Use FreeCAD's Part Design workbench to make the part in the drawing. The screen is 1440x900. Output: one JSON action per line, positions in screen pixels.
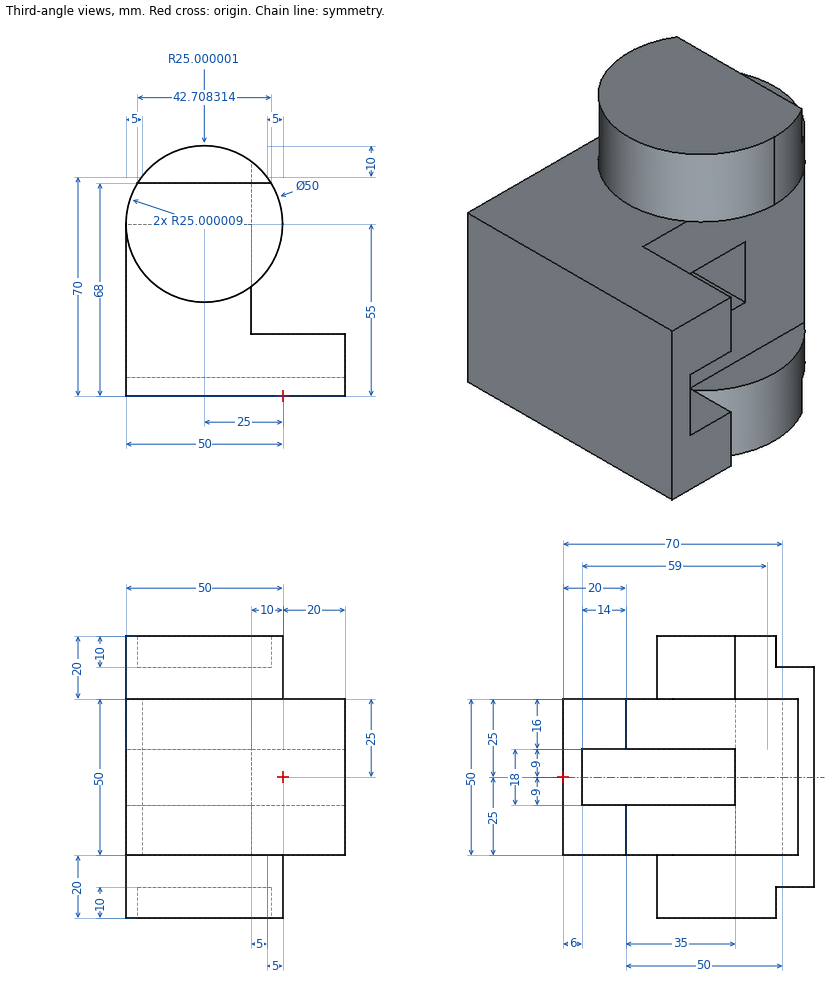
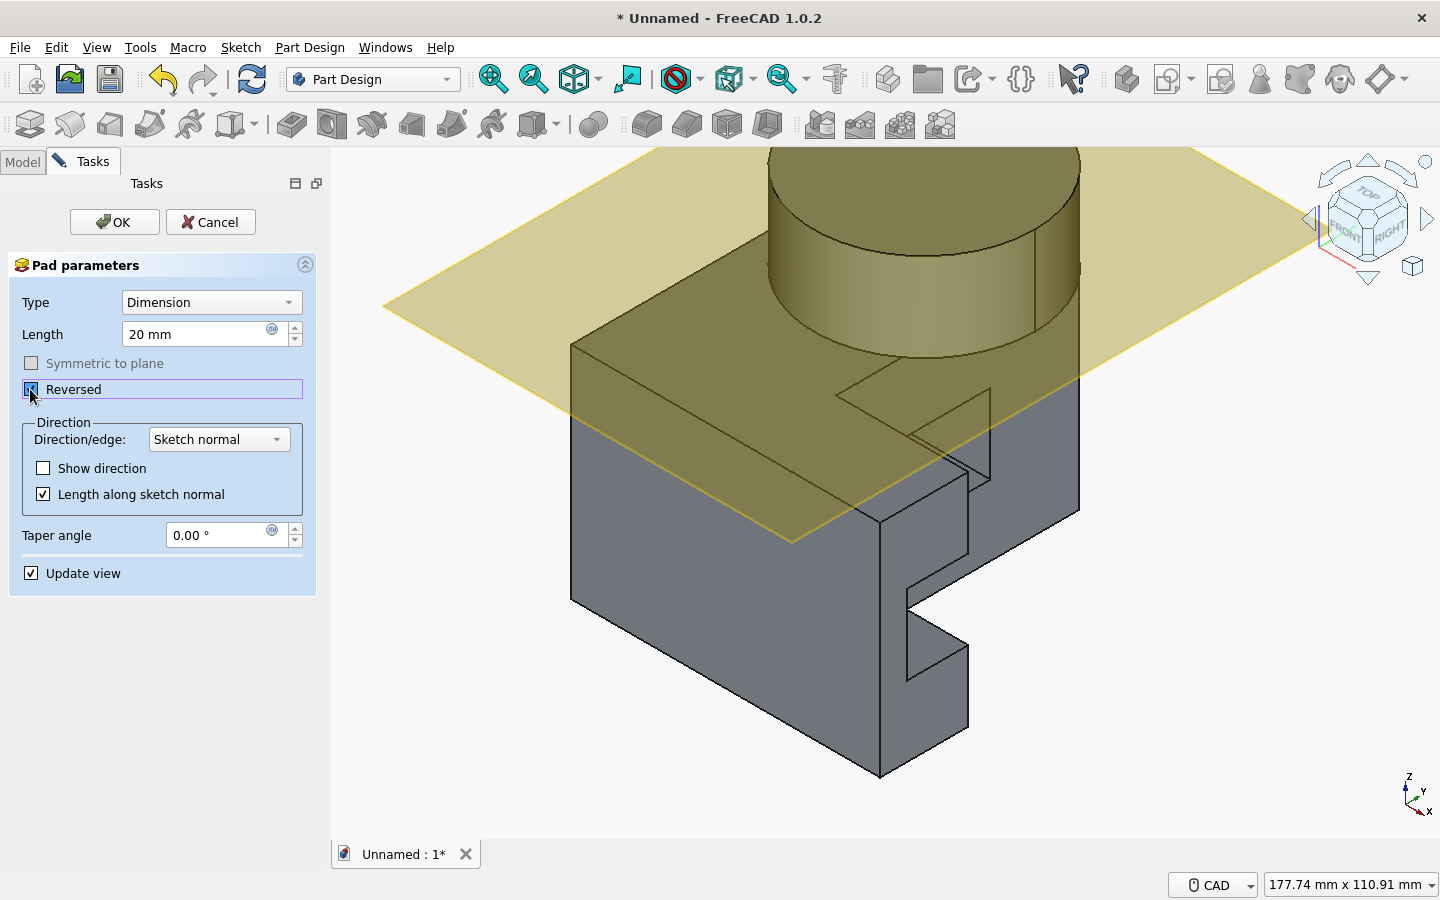
{"action": "left_click", "coordinate": [115, 222]}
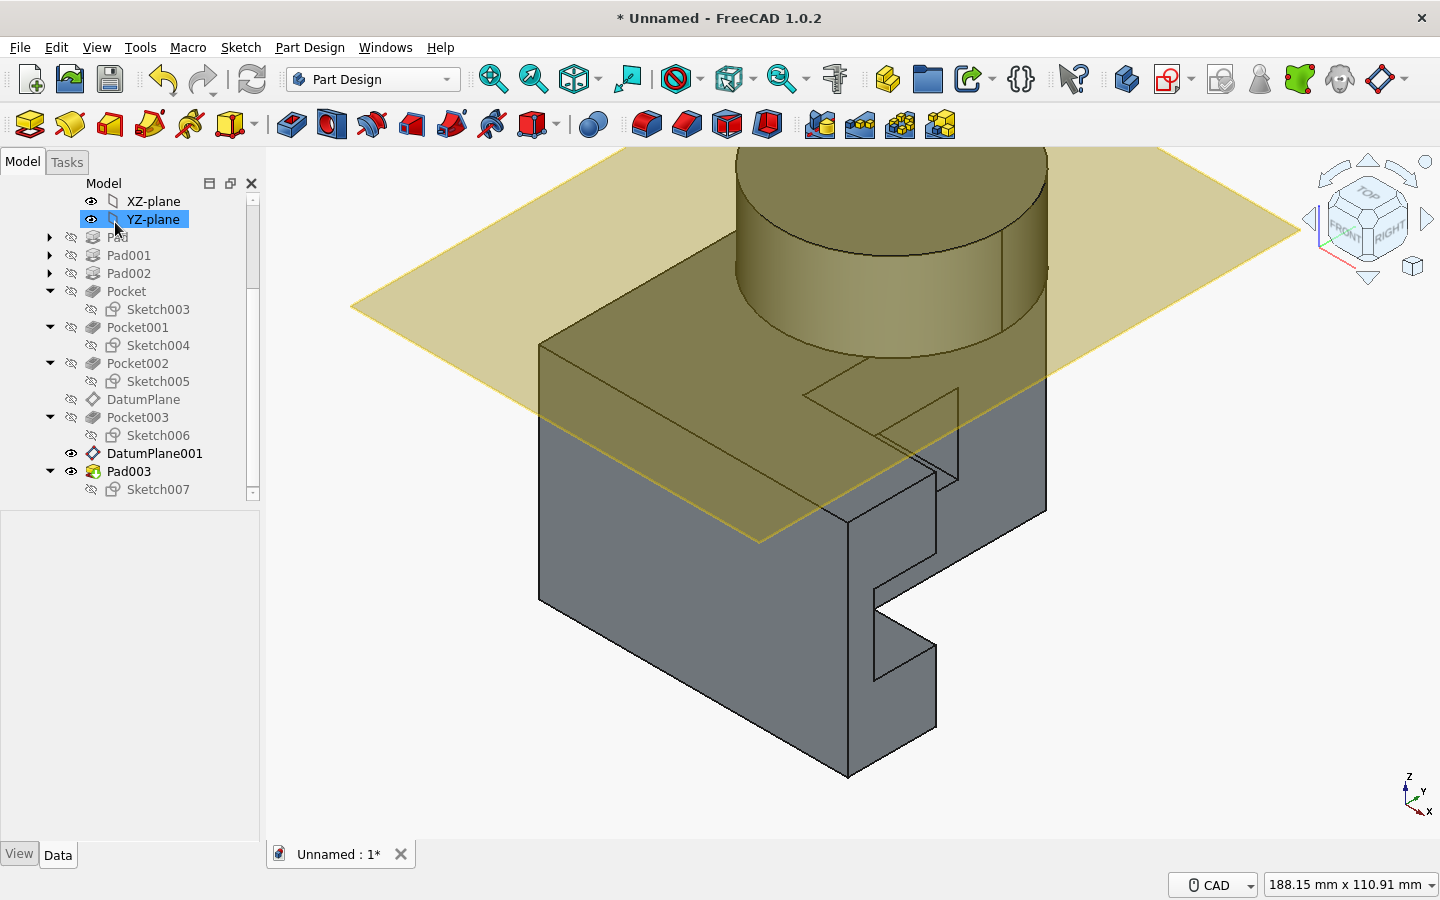
{"action": "left_click", "coordinate": [116, 453]}
{"action": "key", "text": "space"}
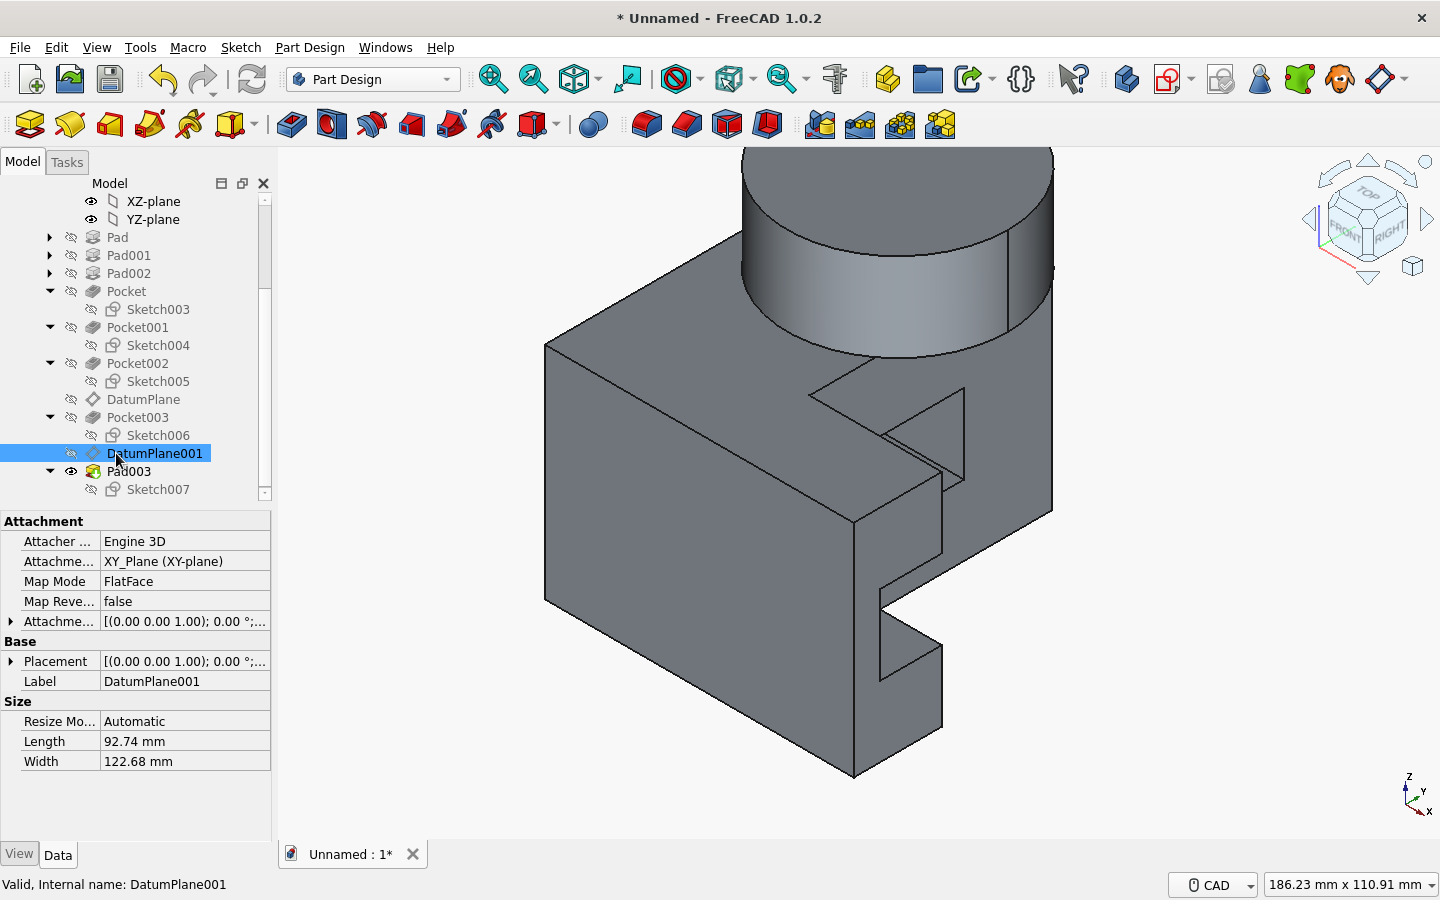
{"action": "left_click", "coordinate": [494, 80]}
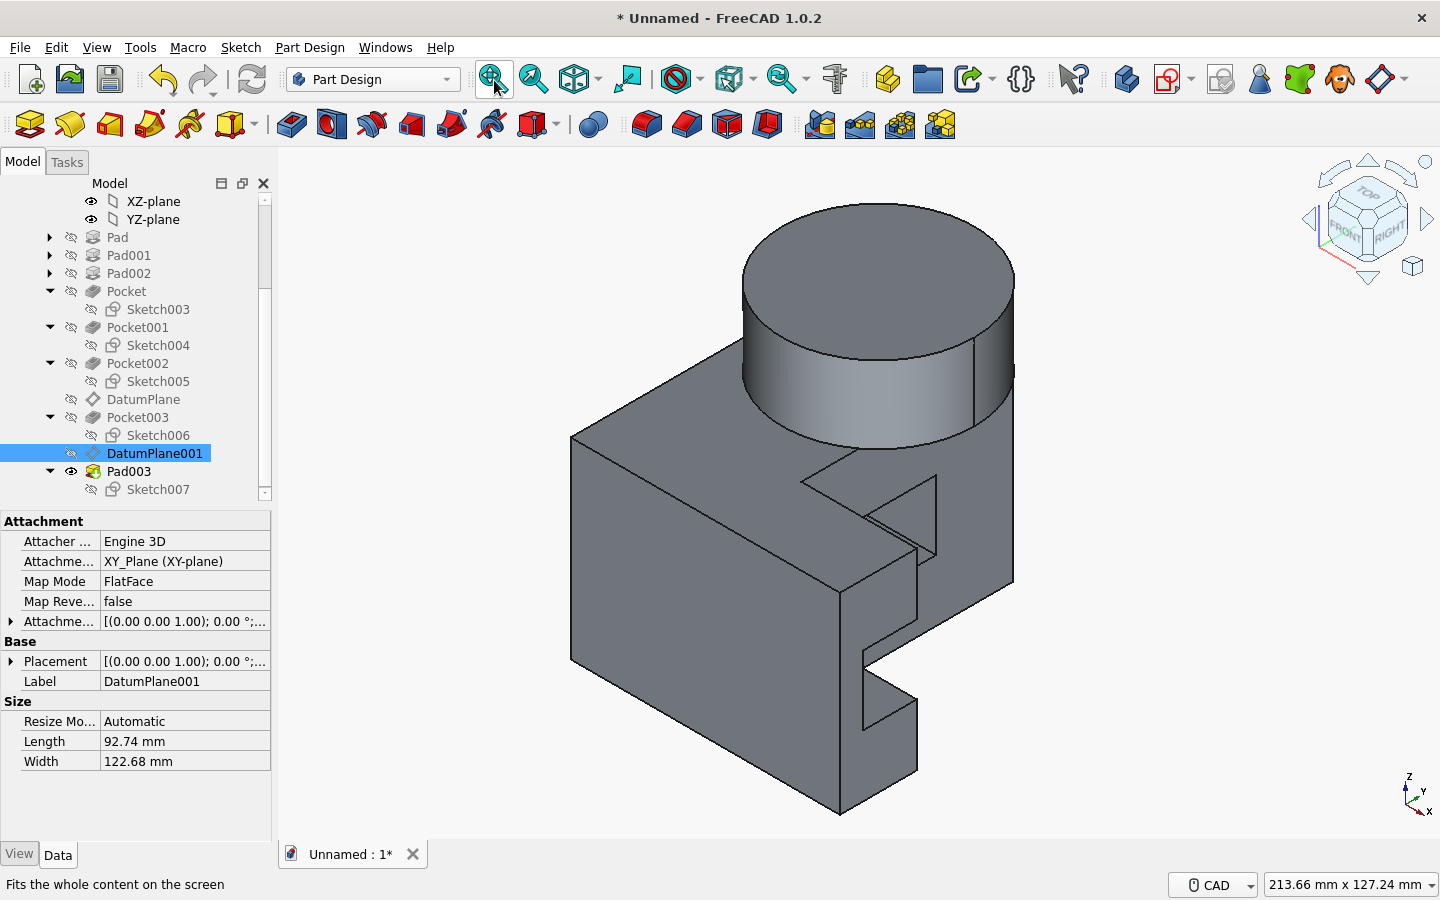
{"action": "key", "text": "5"}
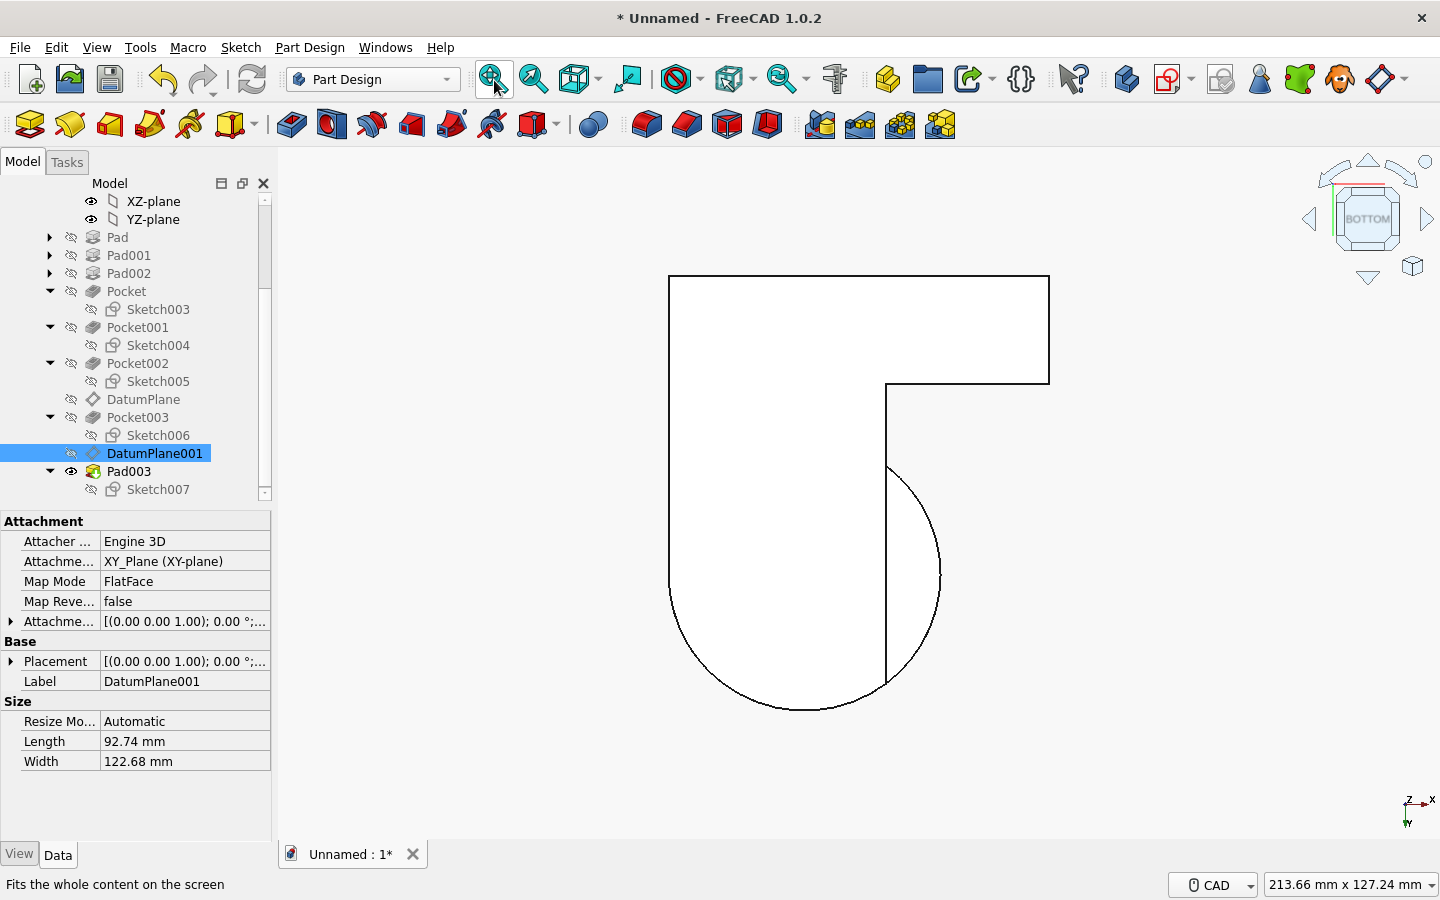
{"action": "left_click", "coordinate": [805, 368]}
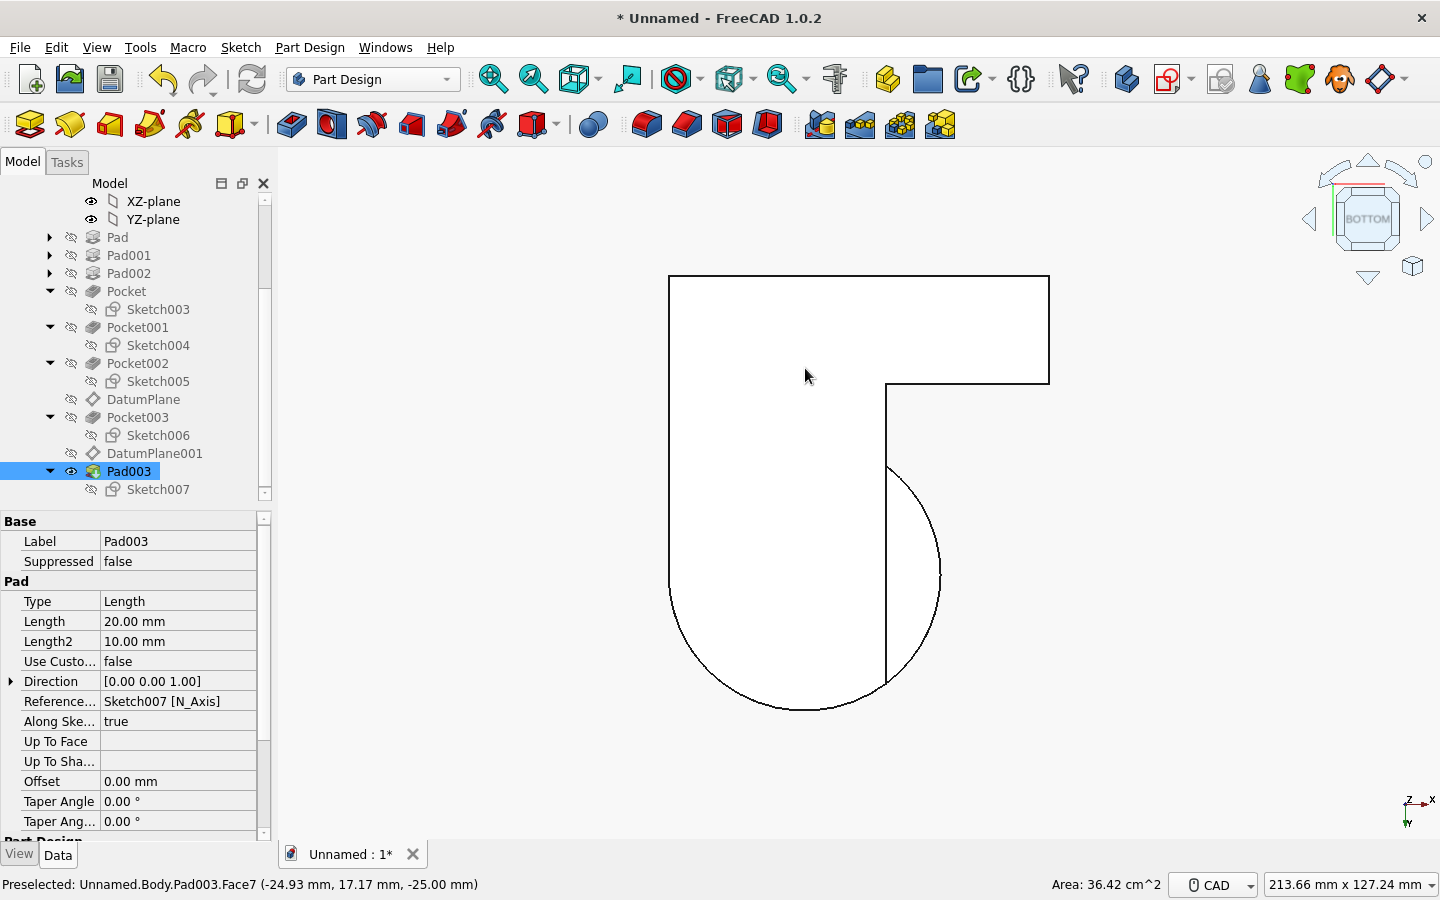
{"action": "left_click", "coordinate": [1168, 80]}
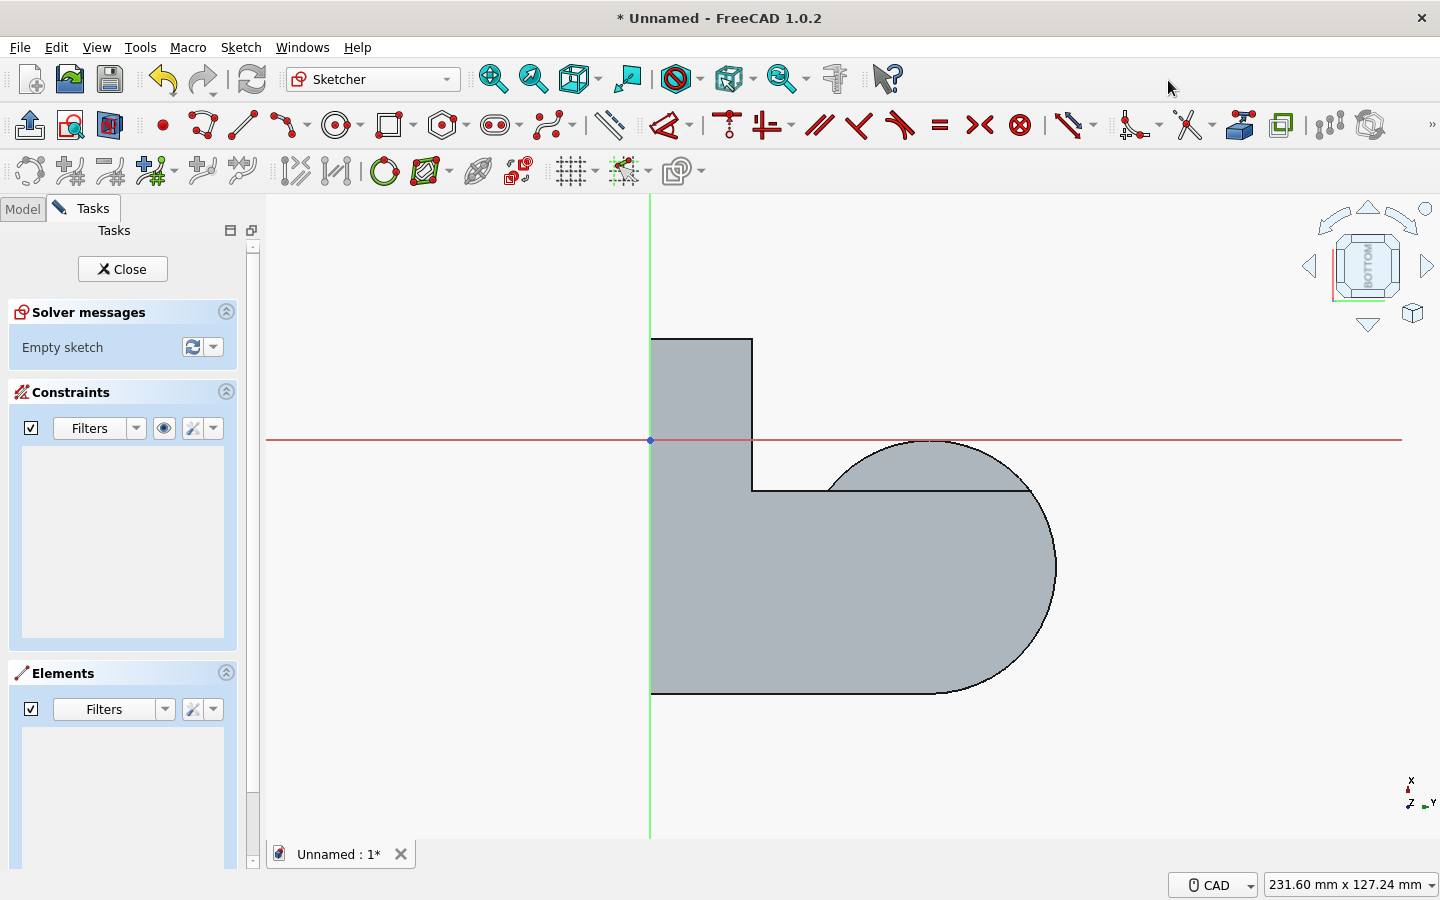
{"action": "scroll", "coordinate": [993, 670], "scroll_direction": "up", "scroll_amount": 2}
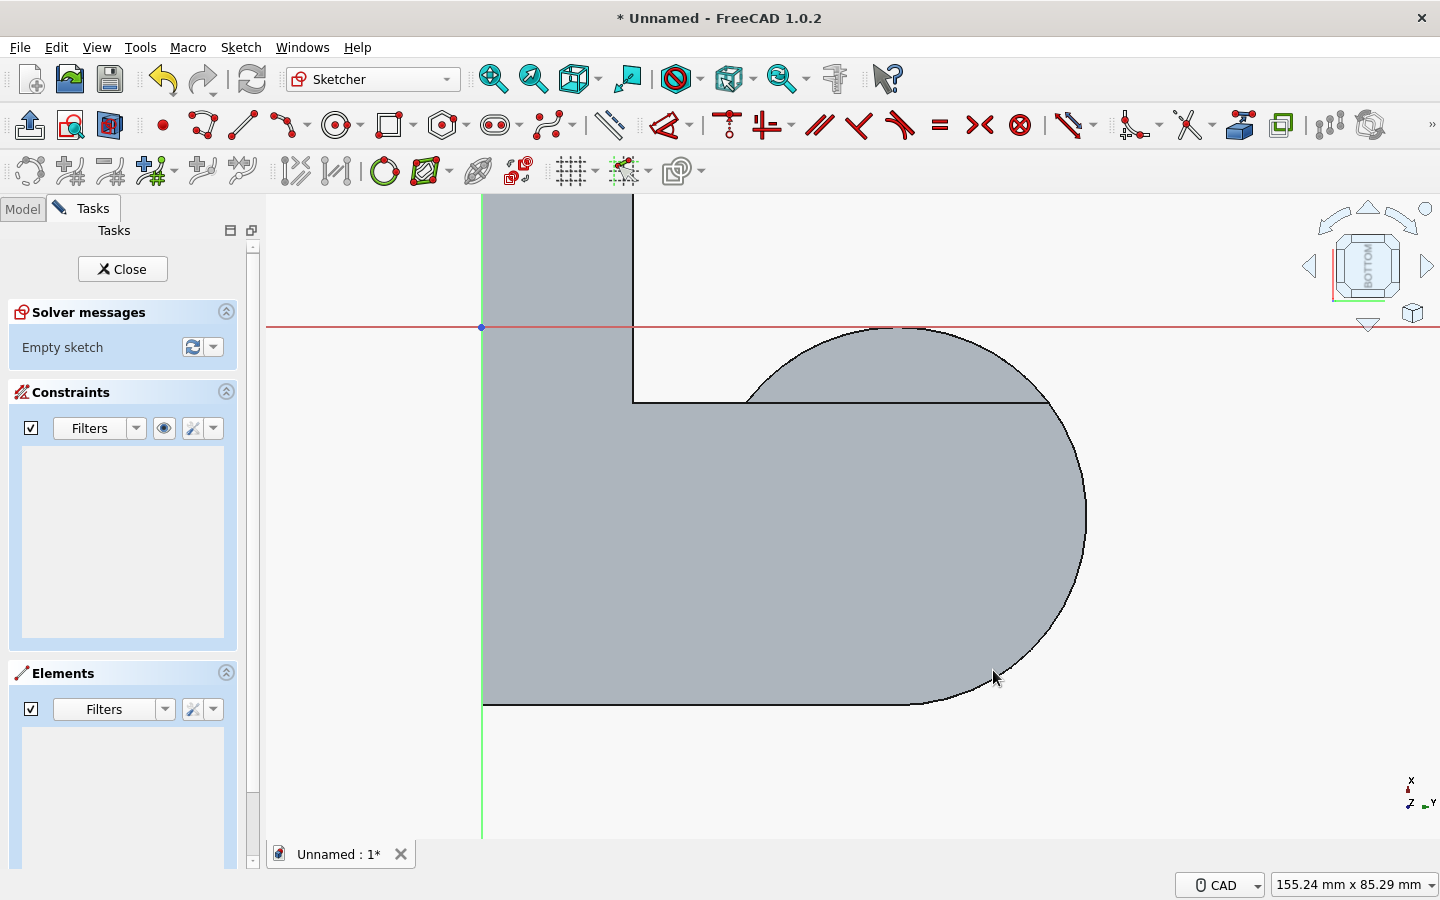
{"action": "left_click", "coordinate": [336, 126]}